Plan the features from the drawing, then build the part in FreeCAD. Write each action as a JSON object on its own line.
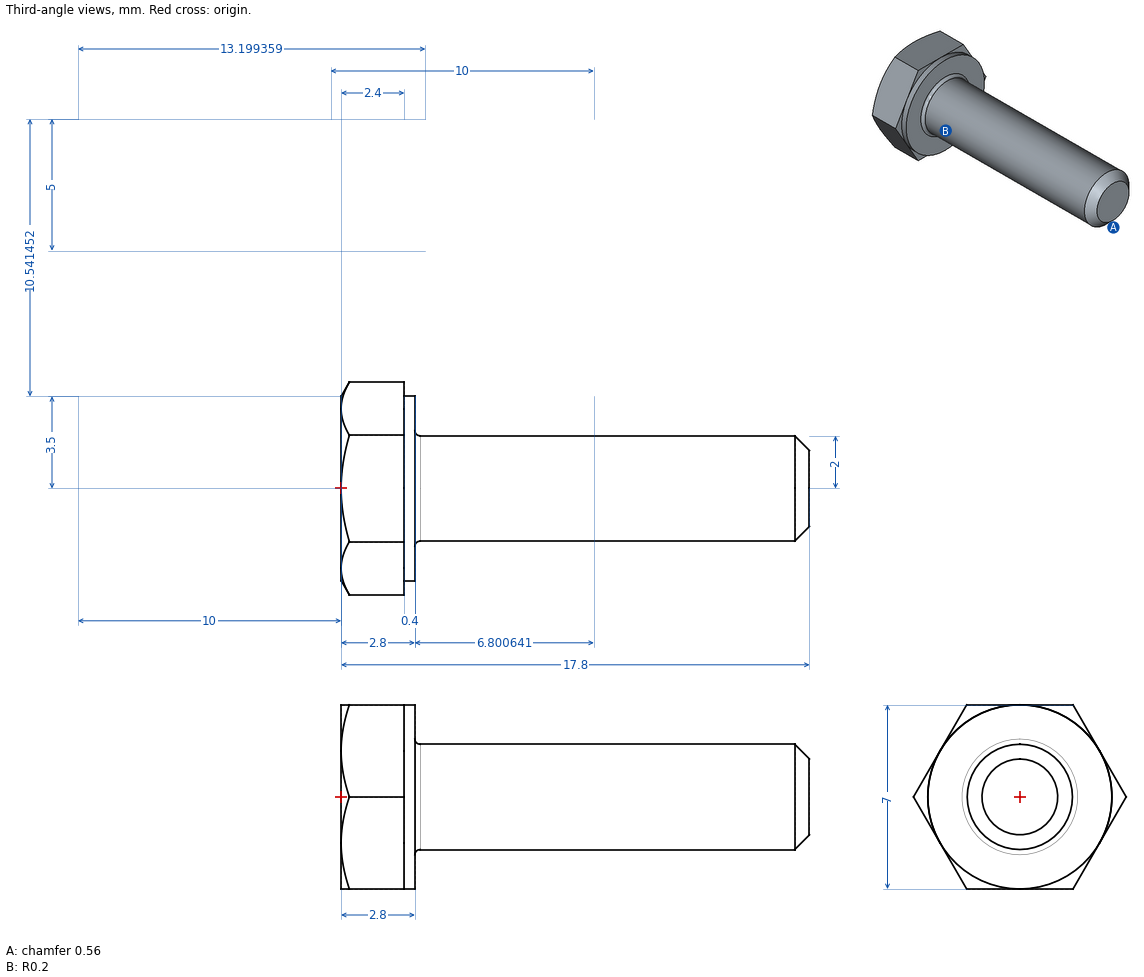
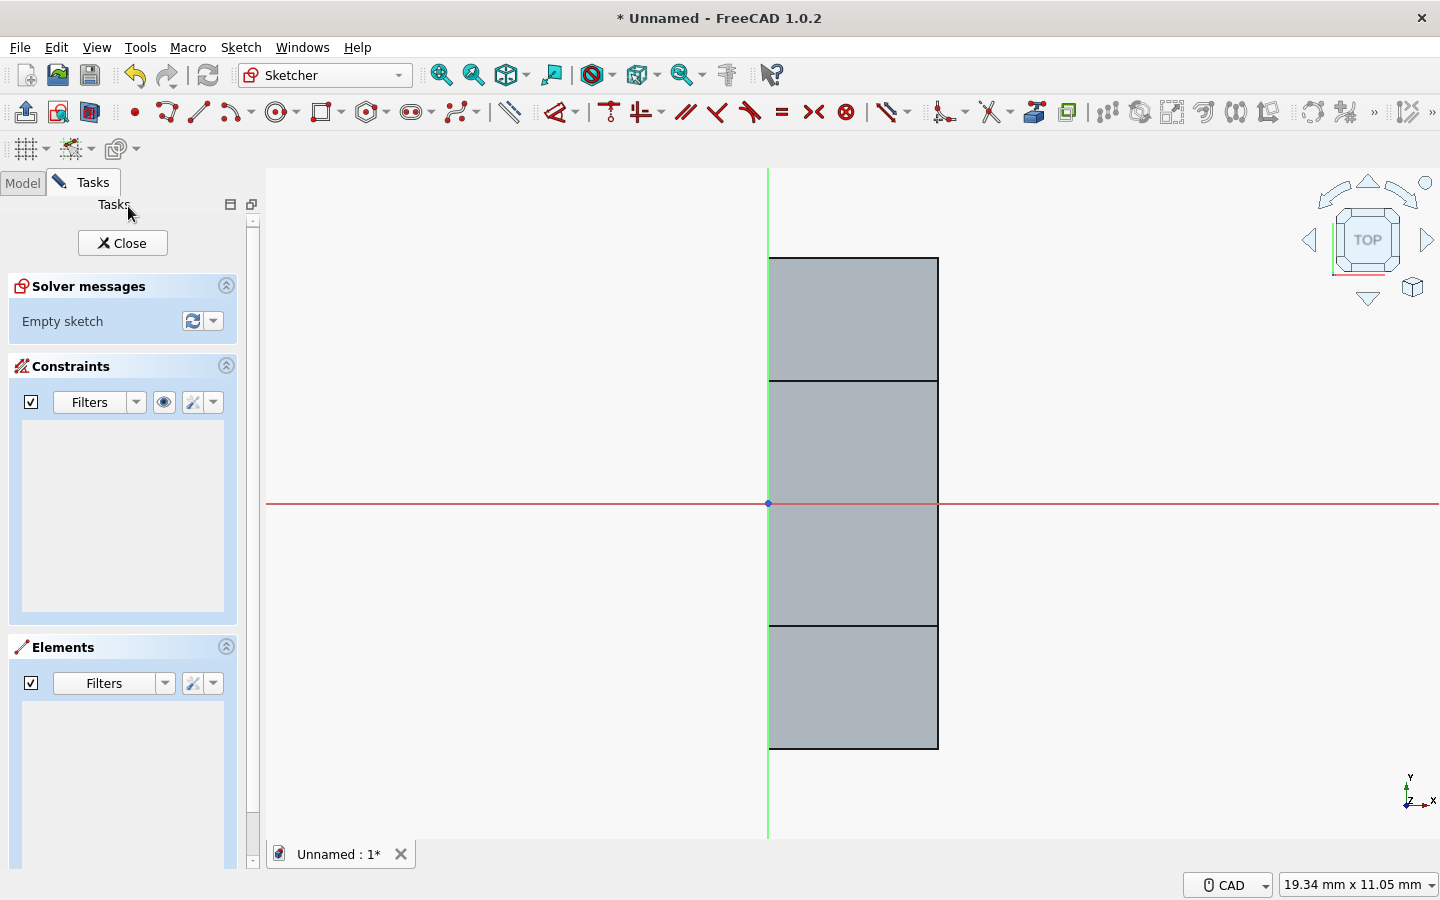
{"action": "scroll", "coordinate": [294, 577], "scroll_direction": "down", "scroll_amount": 3}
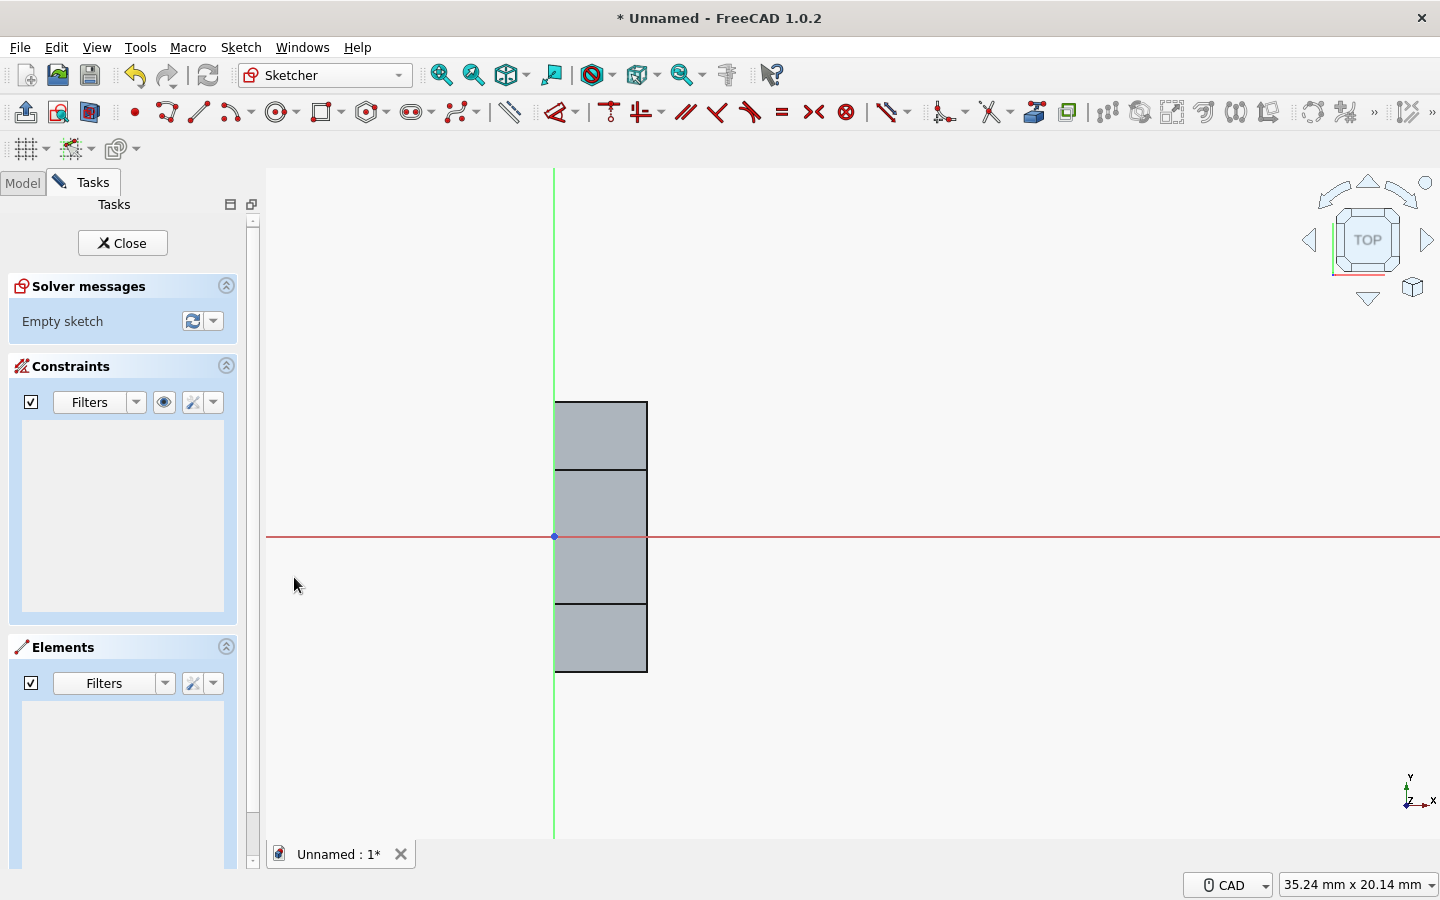
{"action": "left_click", "coordinate": [322, 112]}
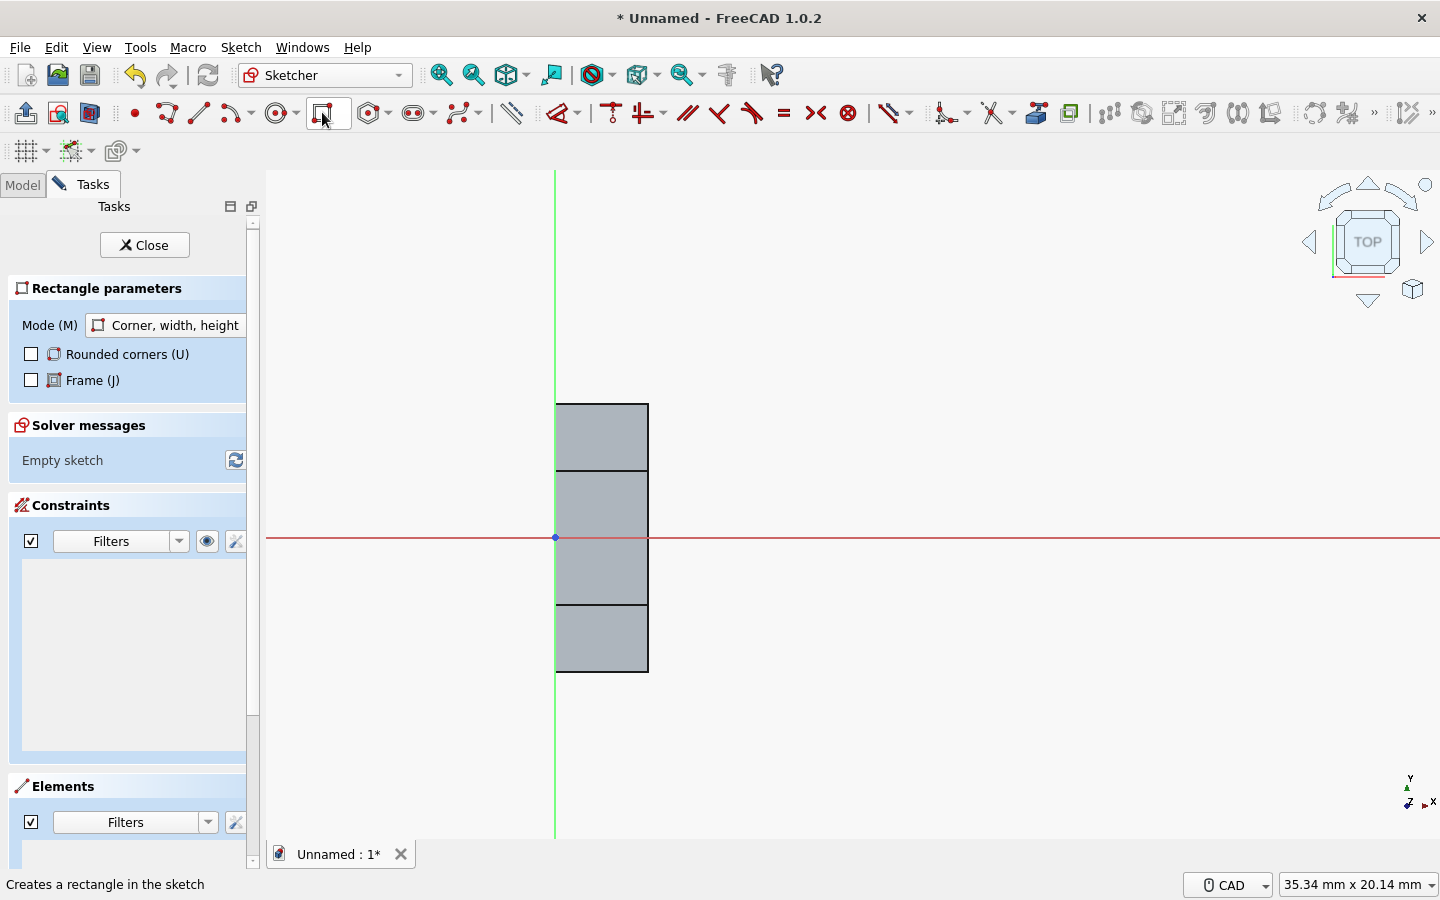
{"action": "left_click", "coordinate": [555, 538]}
{"action": "left_click", "coordinate": [1146, 471]}
{"action": "key", "text": "Escape"}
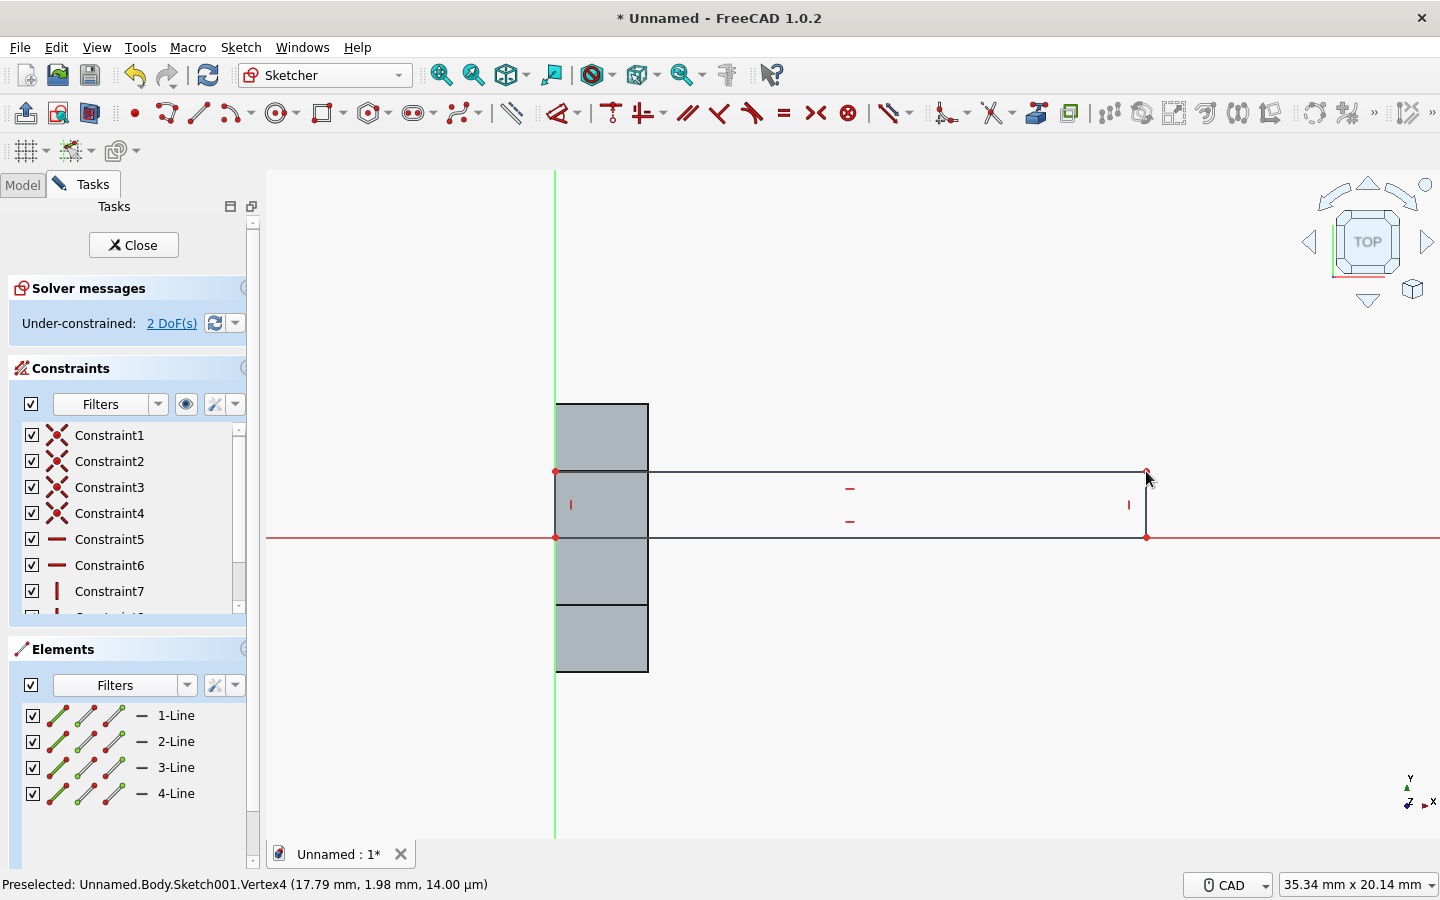
{"action": "key", "text": "d"}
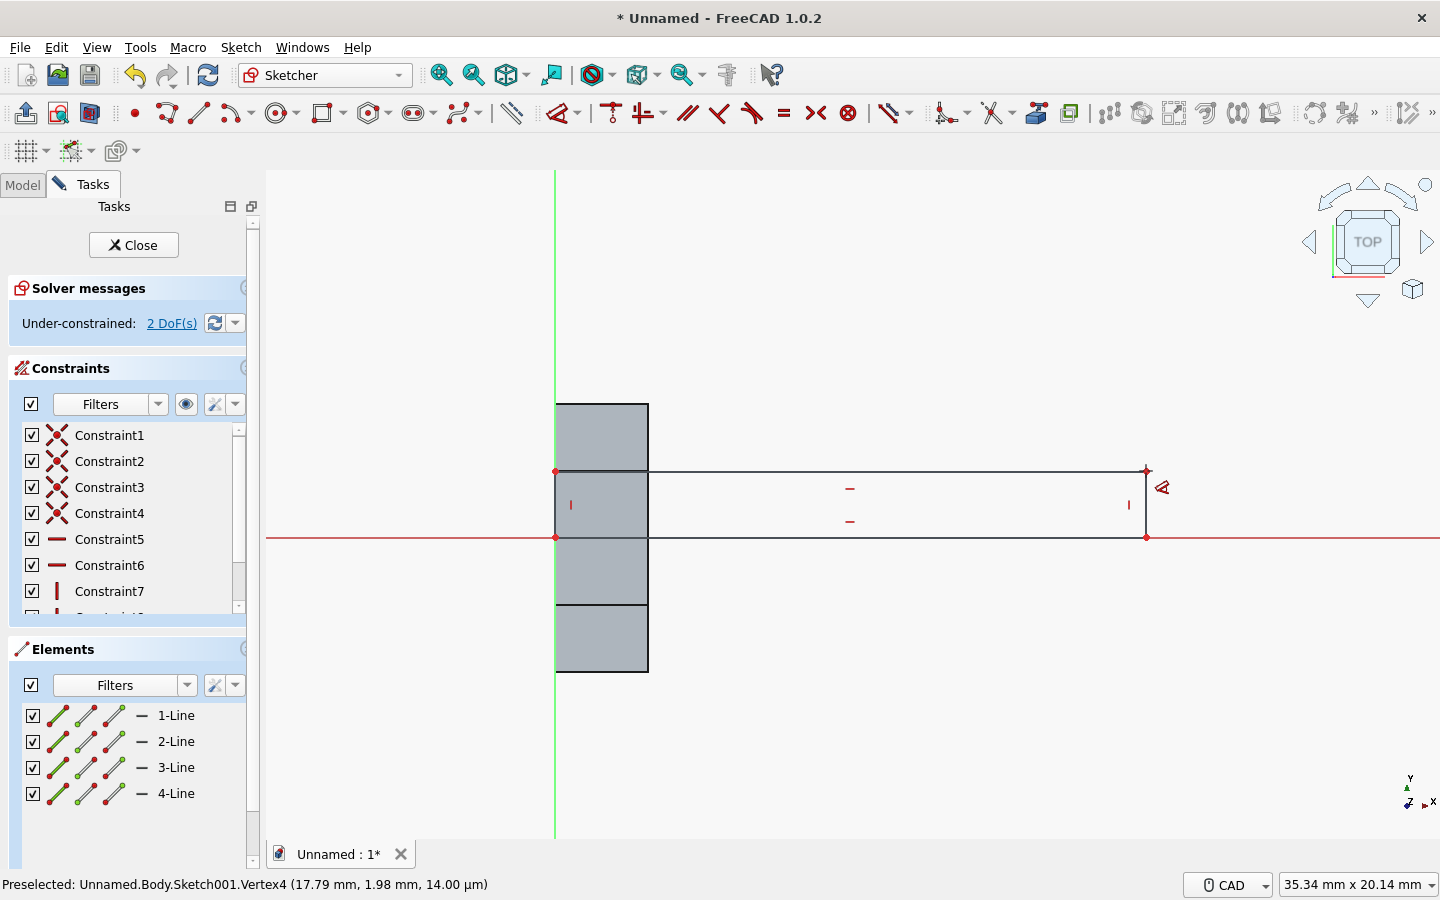
{"action": "left_click", "coordinate": [1146, 518]}
{"action": "left_click", "coordinate": [1180, 505]}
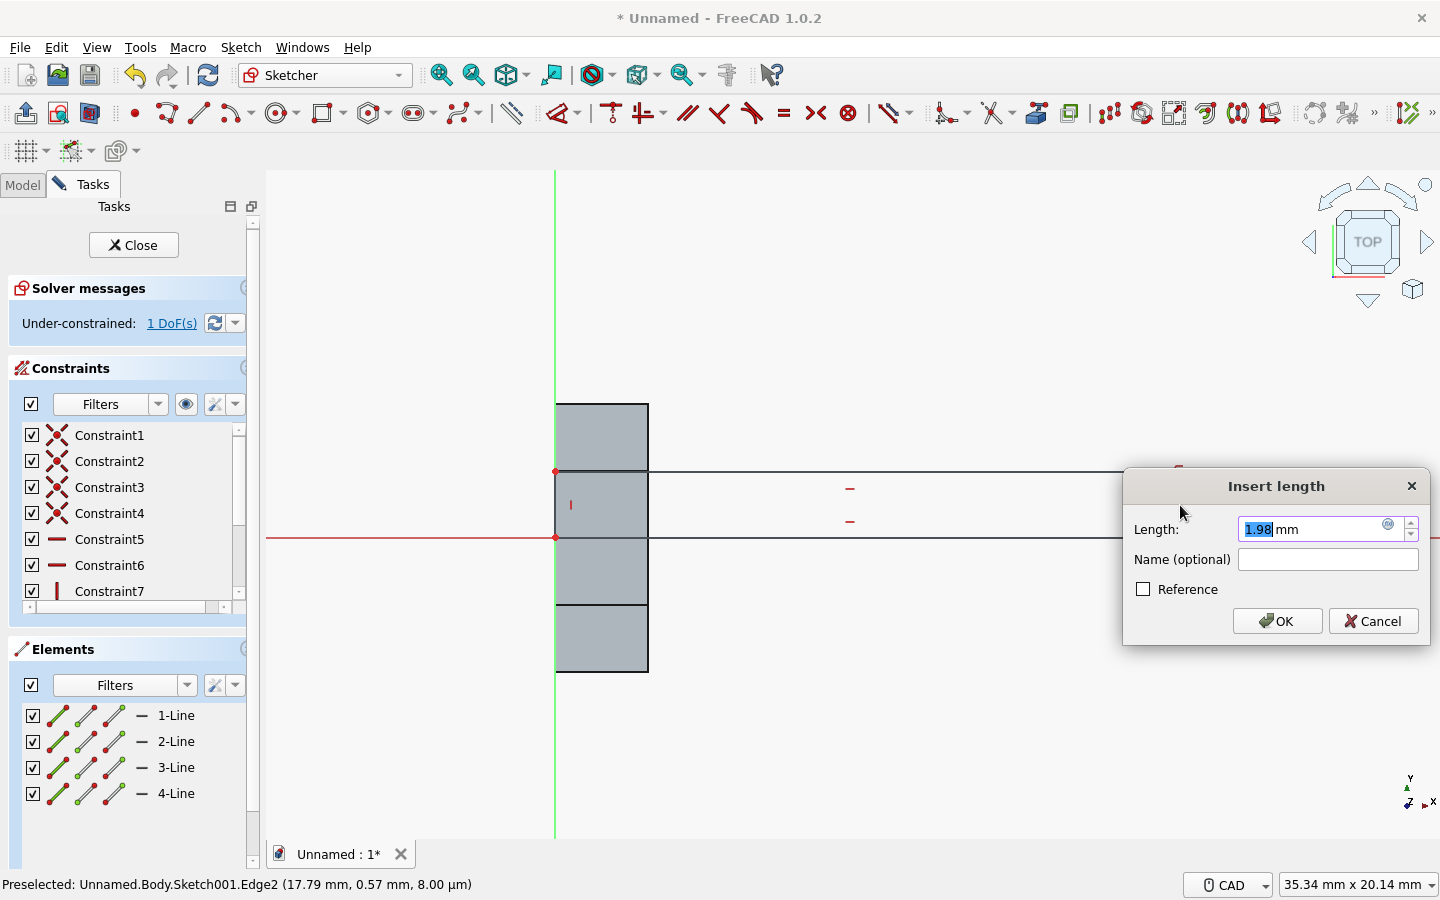
{"action": "type", "text": "2"}
{"action": "key", "text": "Return"}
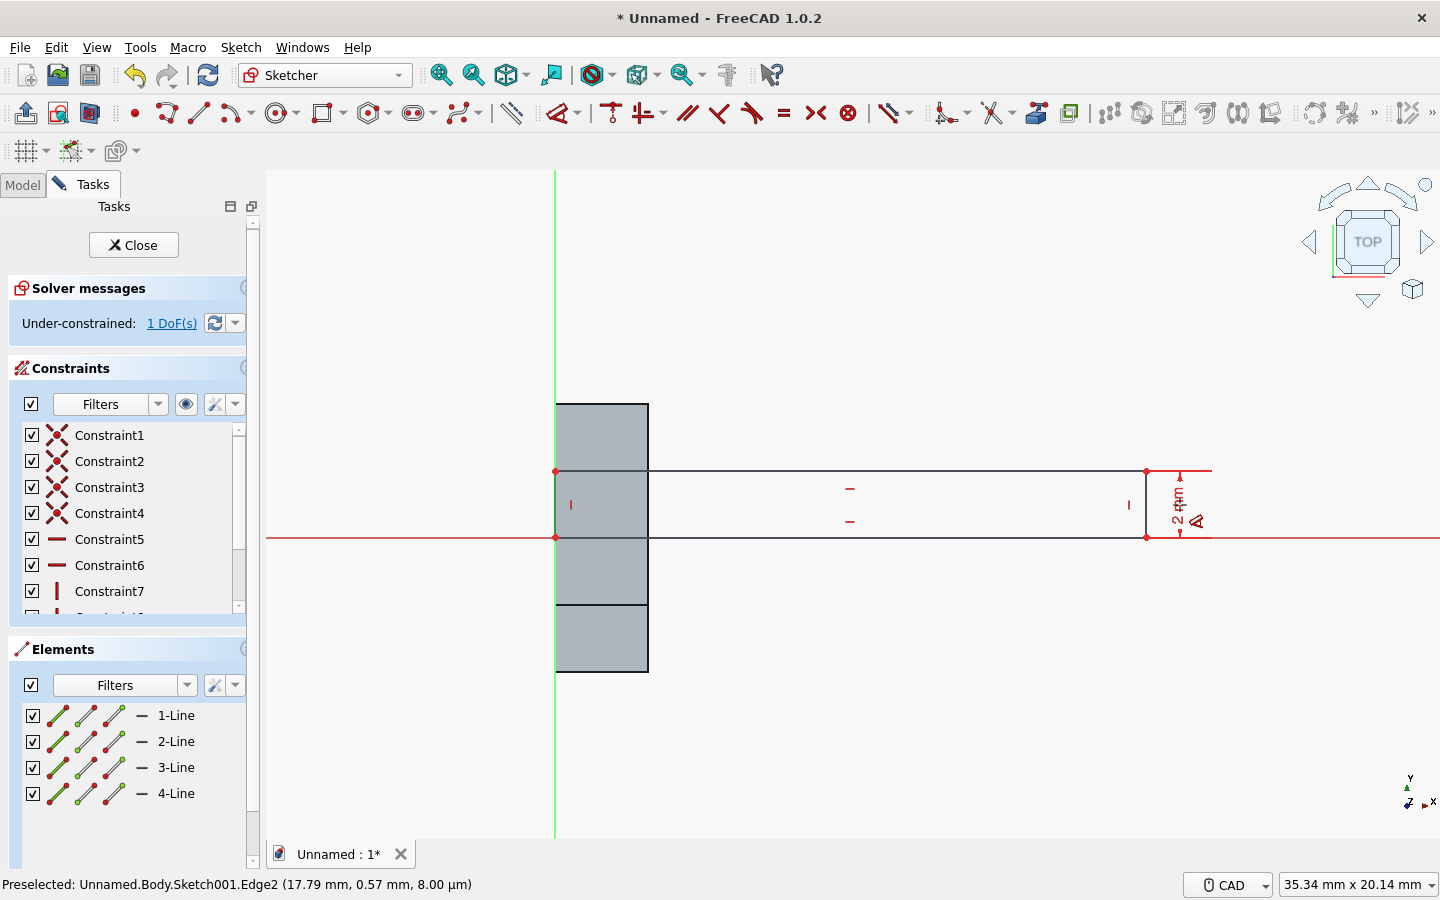
{"action": "left_click", "coordinate": [732, 538]}
{"action": "left_click", "coordinate": [851, 572]}